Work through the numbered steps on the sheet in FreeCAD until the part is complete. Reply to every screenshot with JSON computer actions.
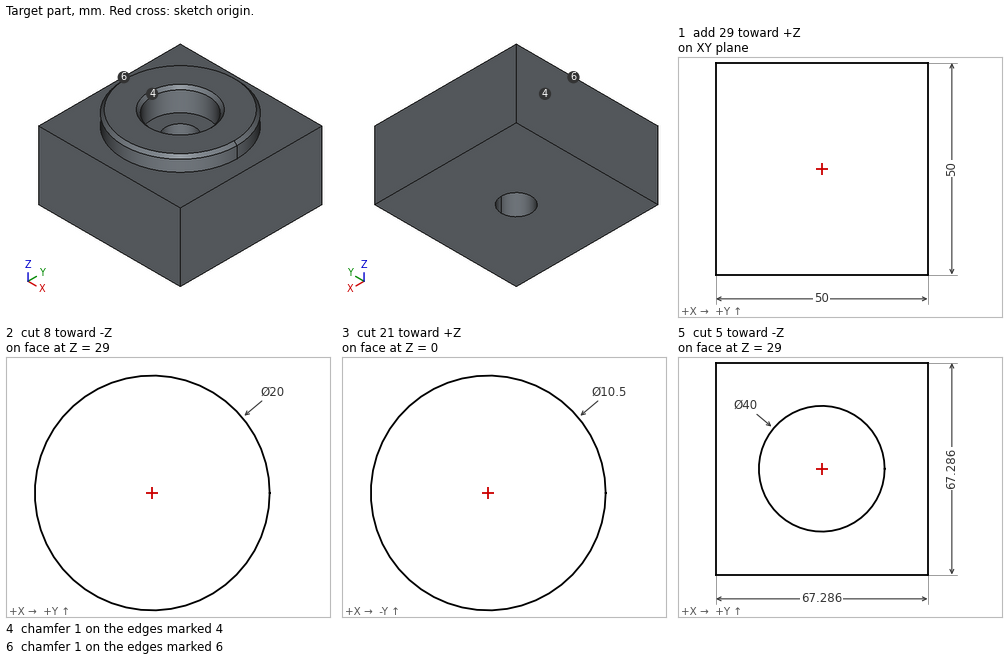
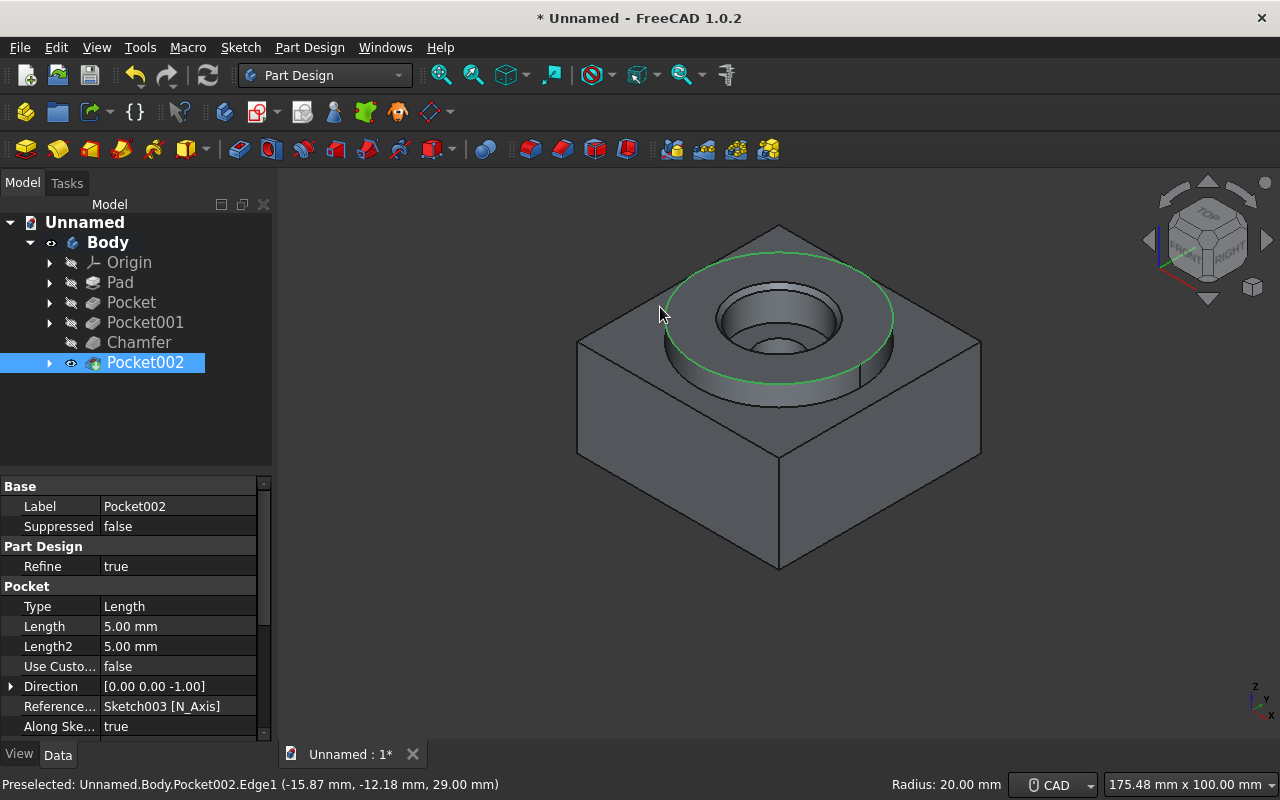
{"action": "left_click", "coordinate": [564, 150]}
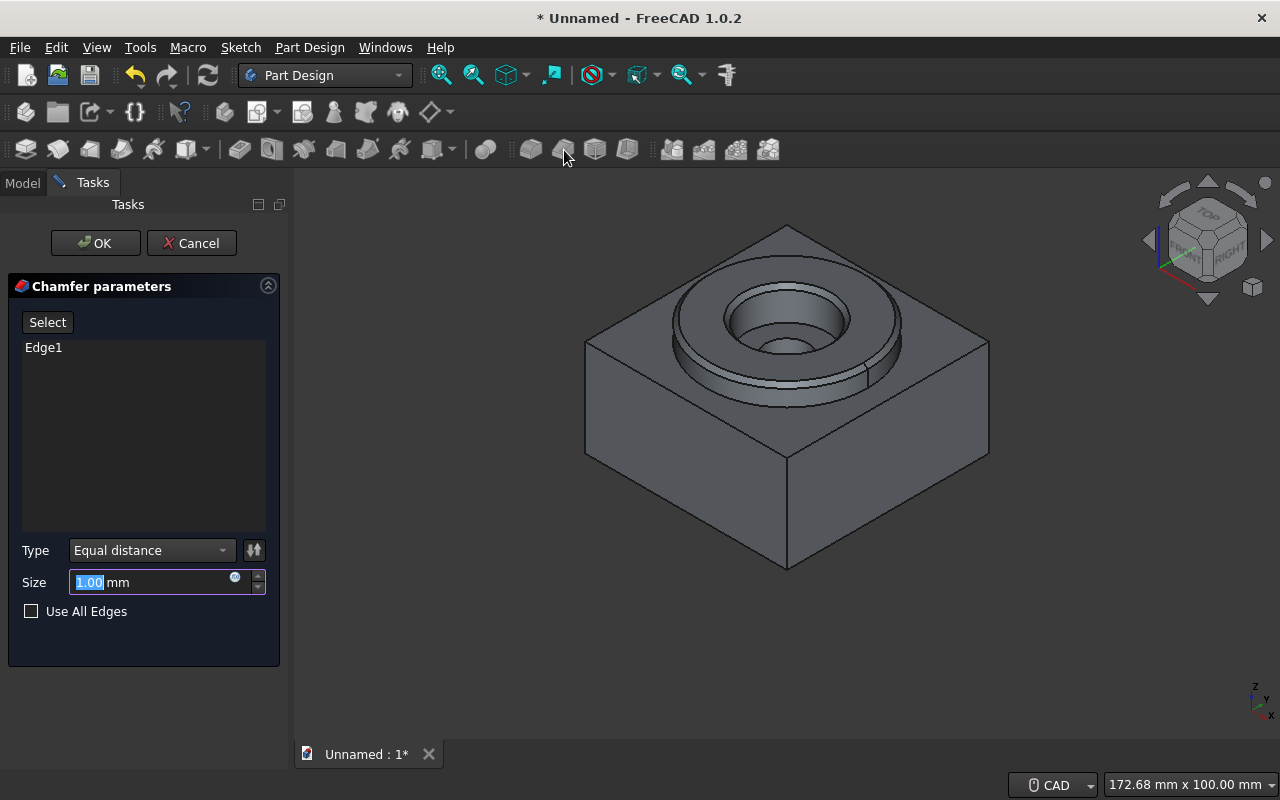
{"action": "type", "text": "1"}
{"action": "key", "text": "Tab"}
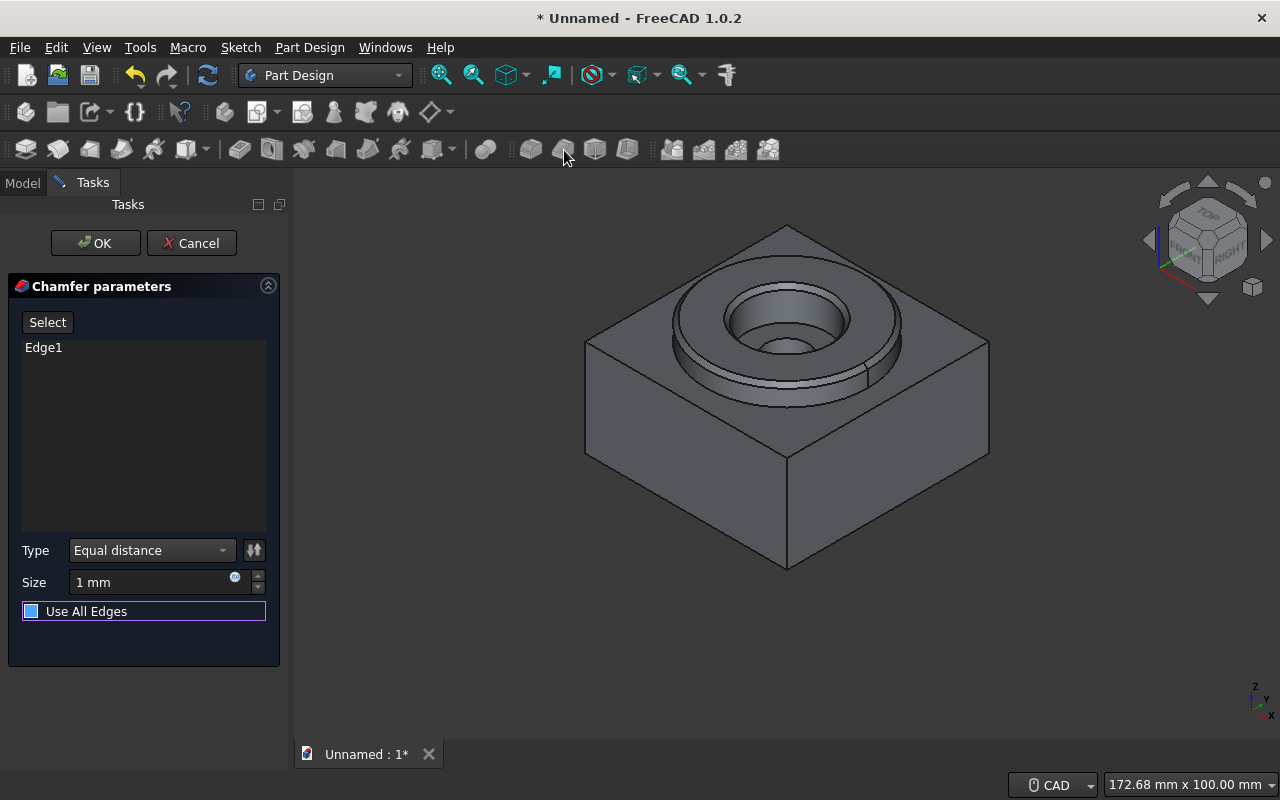
{"action": "left_click", "coordinate": [96, 243]}